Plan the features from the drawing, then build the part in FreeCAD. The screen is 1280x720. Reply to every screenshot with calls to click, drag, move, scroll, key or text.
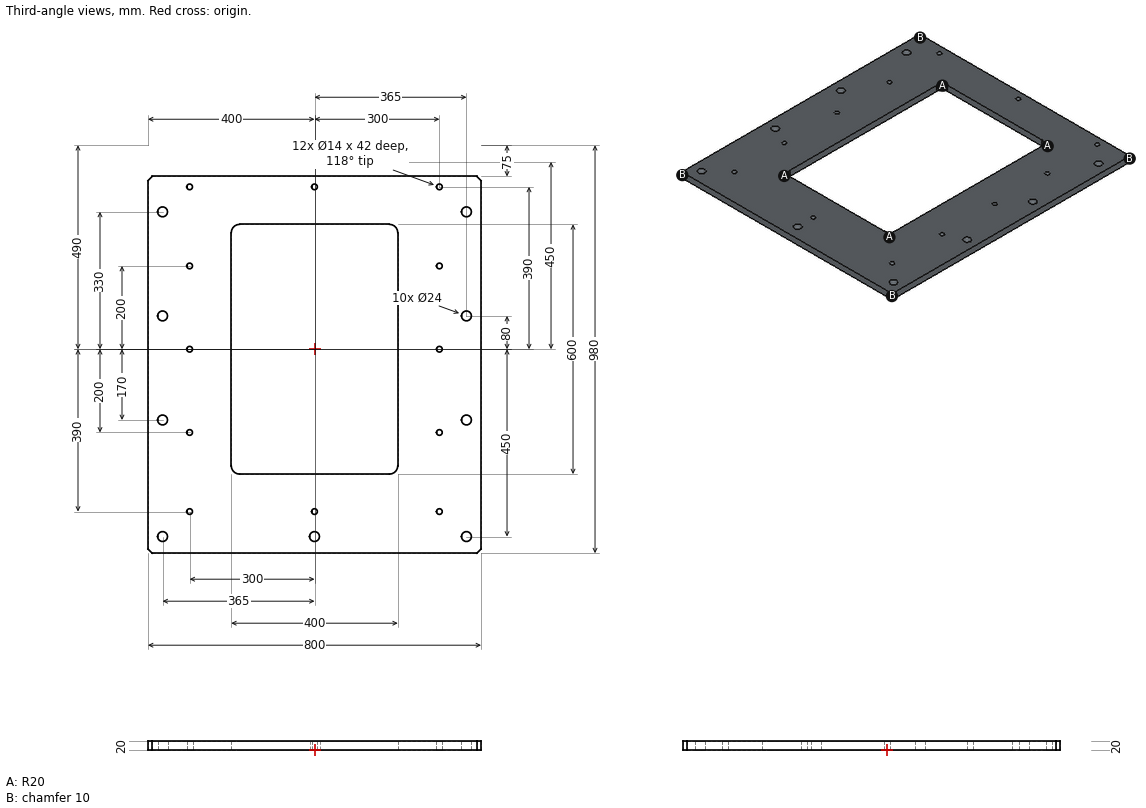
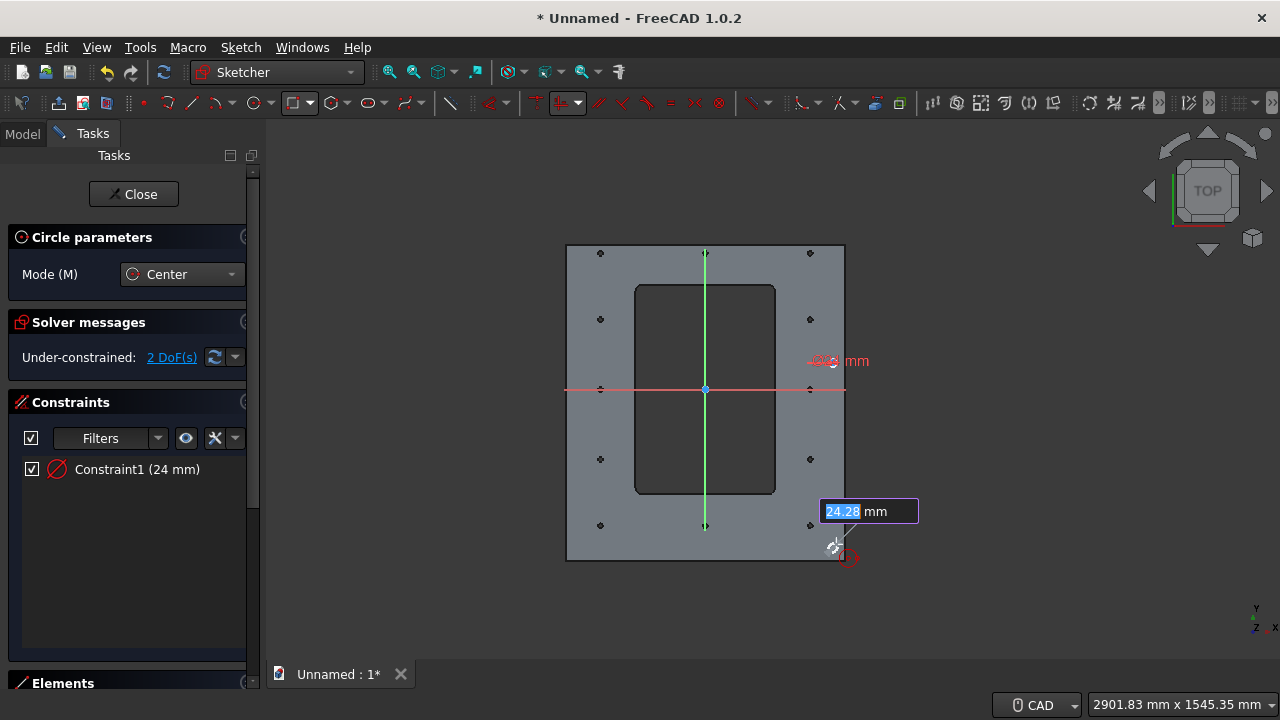
text(24)
key(Return)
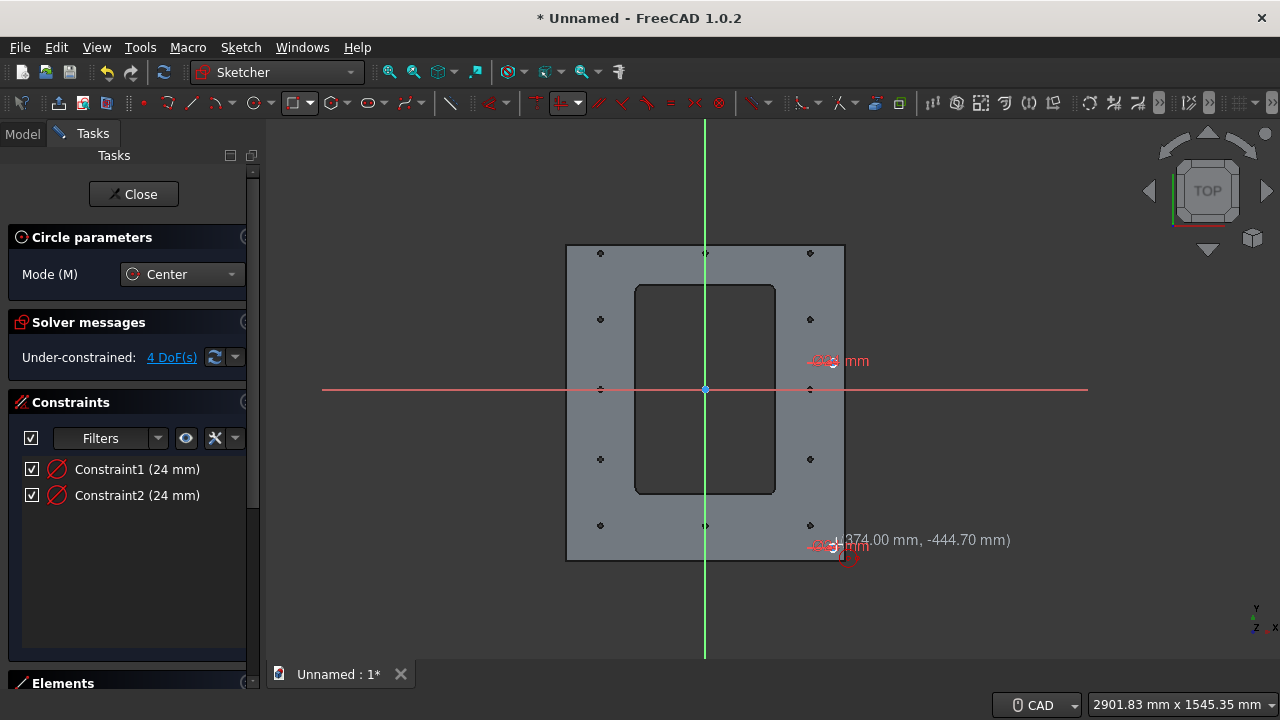
scroll(578, 547, up, 9)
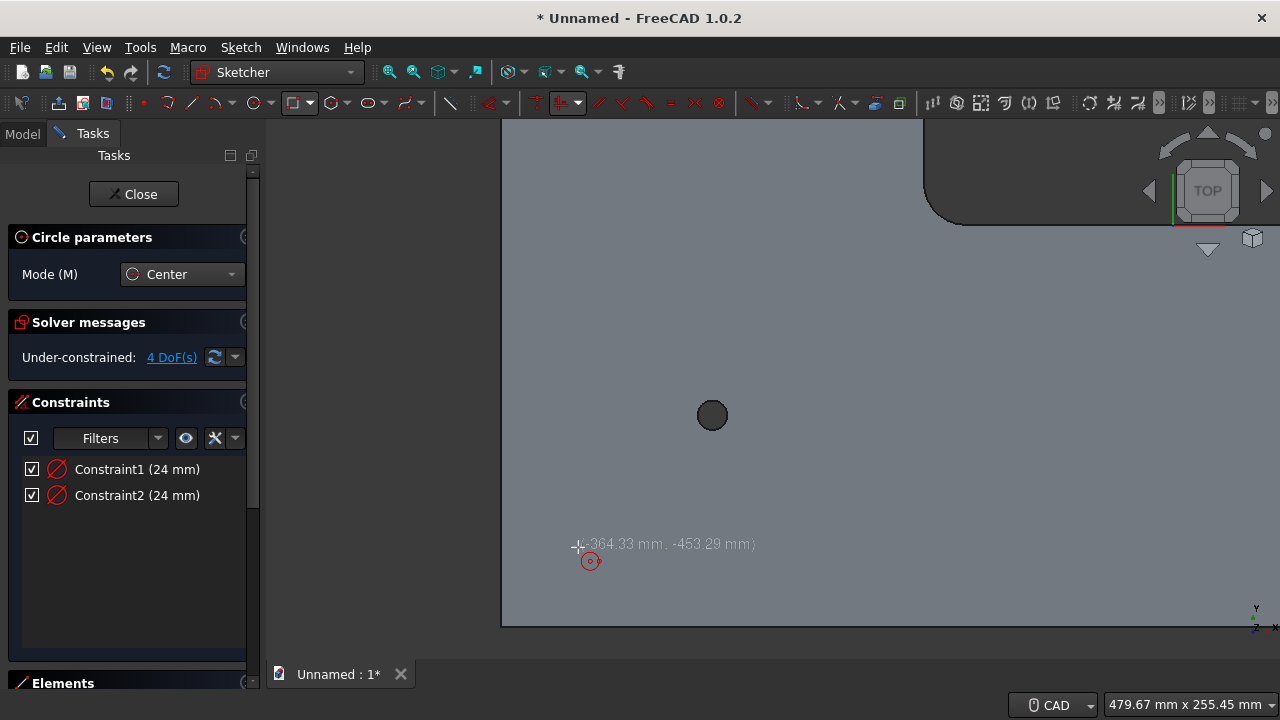
scroll(577, 547, down, 9)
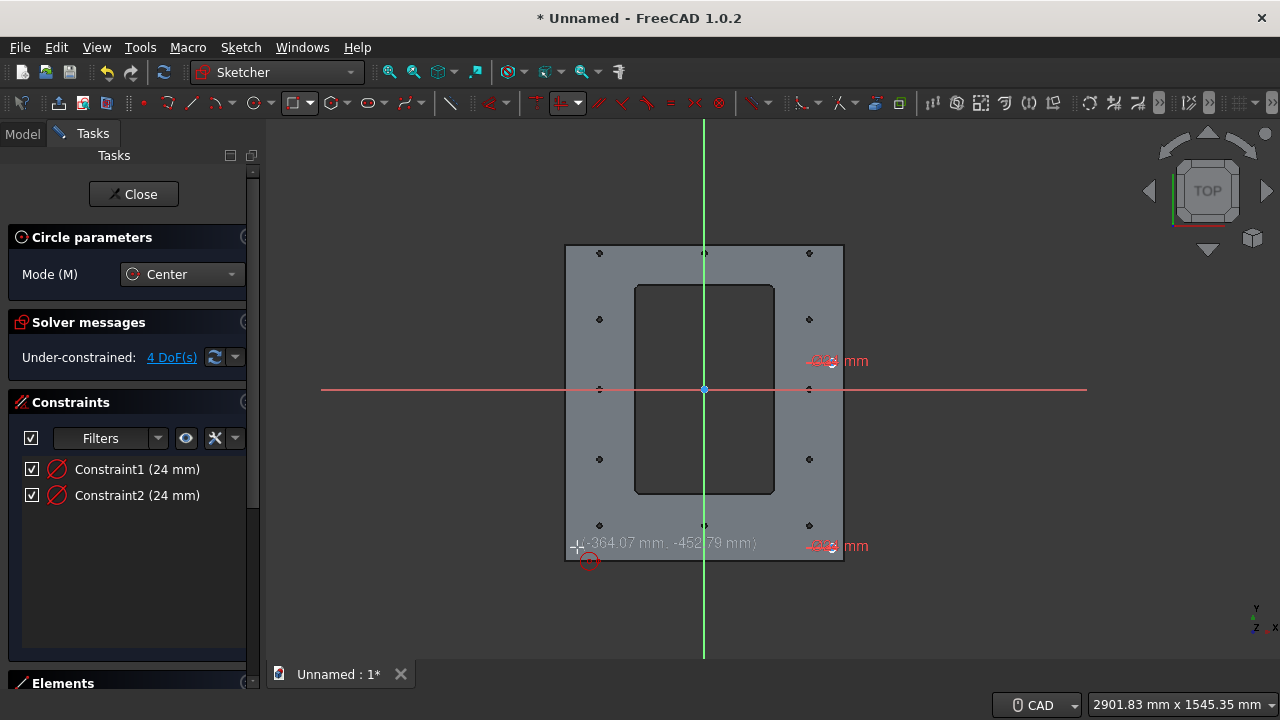
click(577, 547)
move(580, 544)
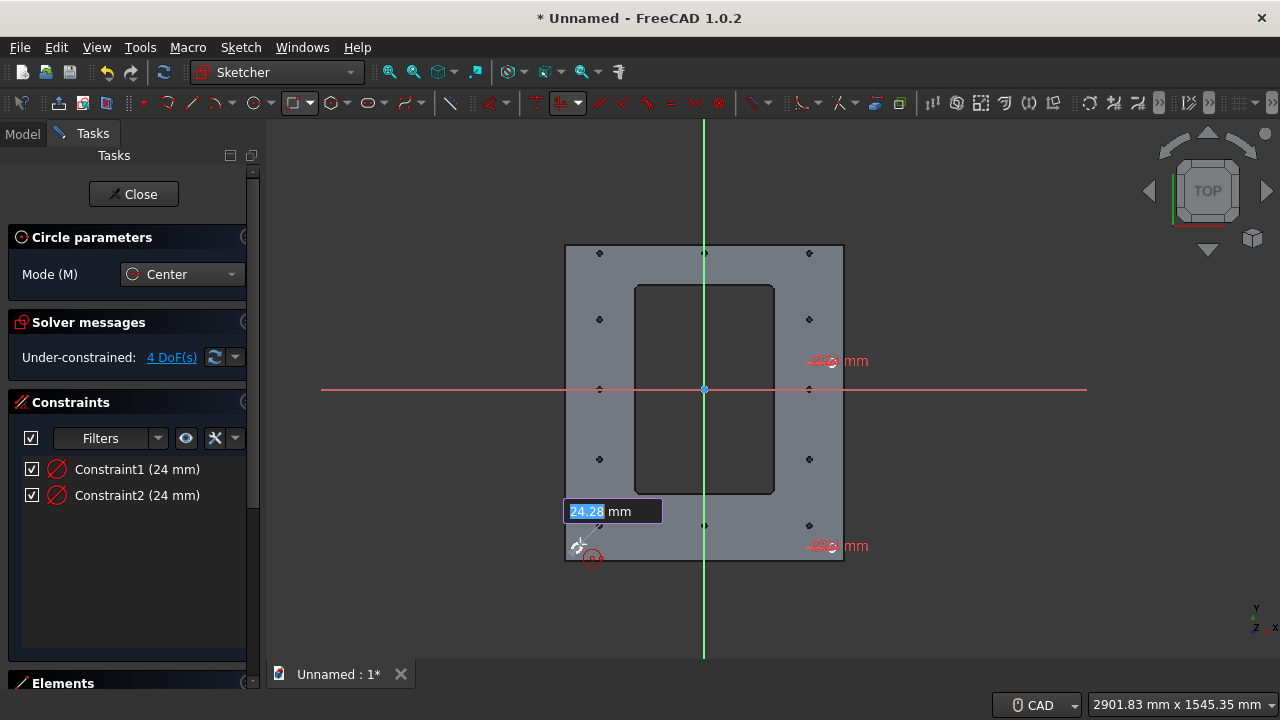
text(24)
key(Return)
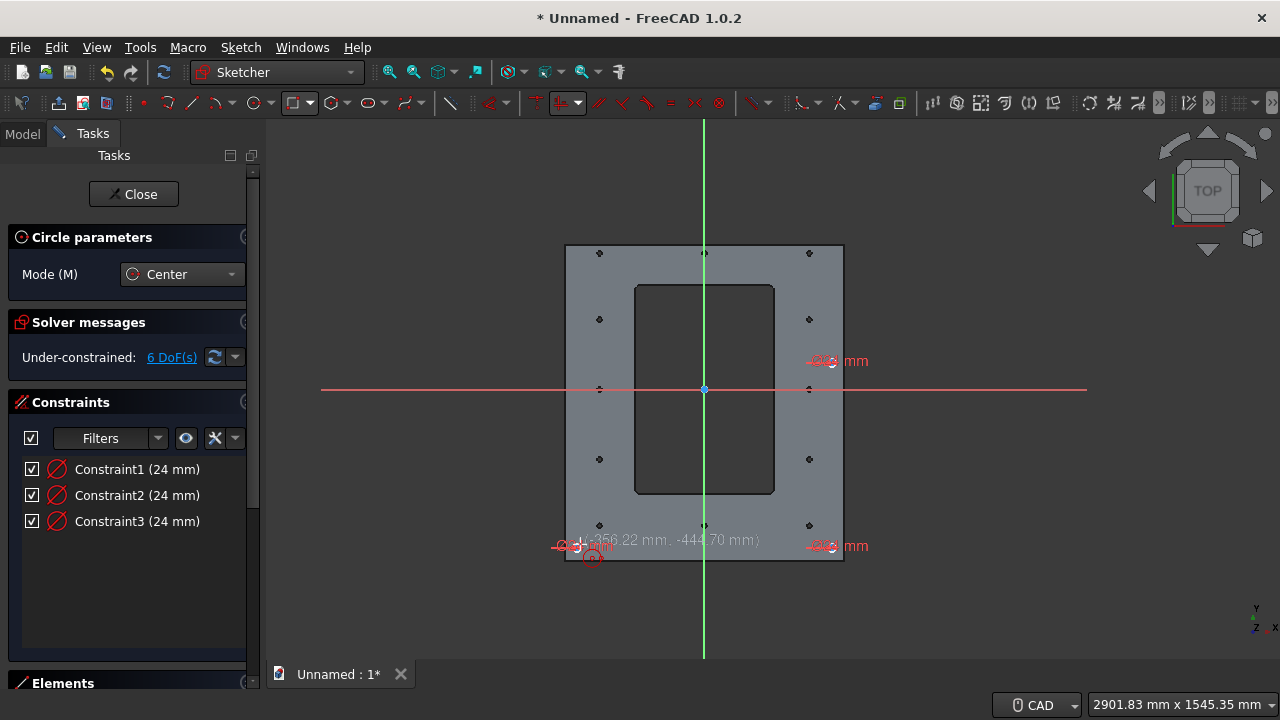
scroll(704, 547, up, 9)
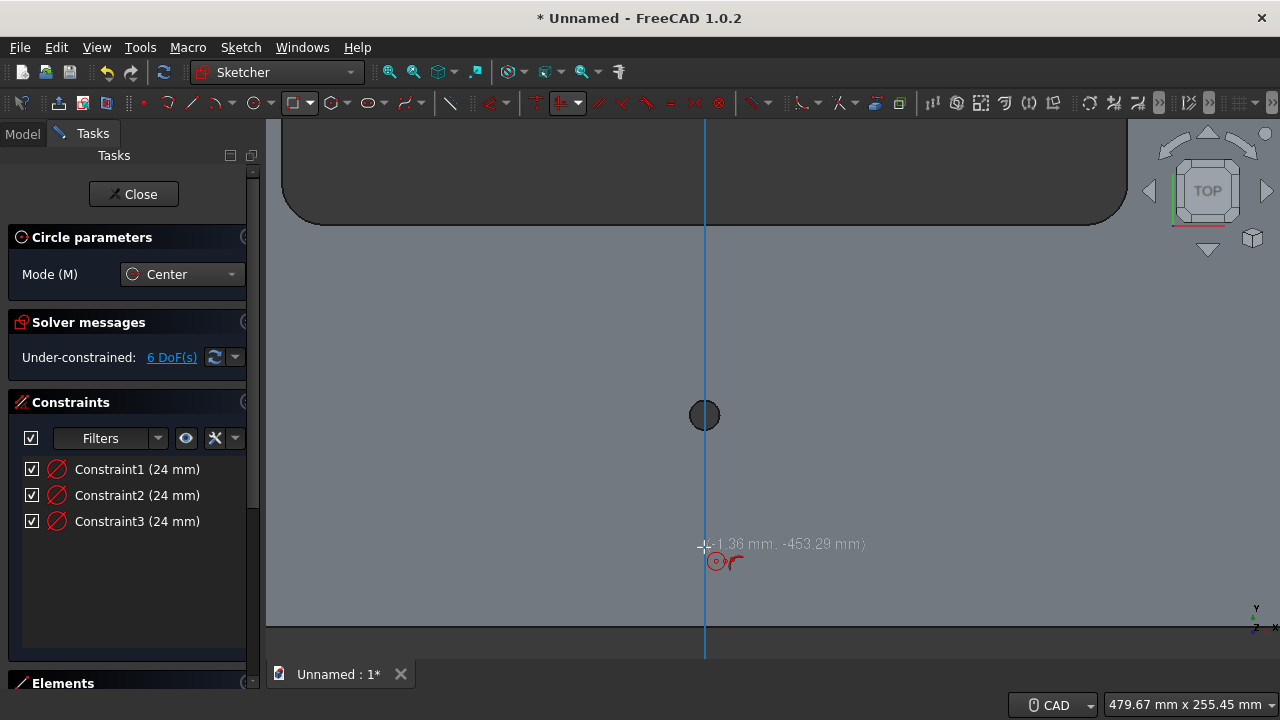
scroll(704, 547, down, 9)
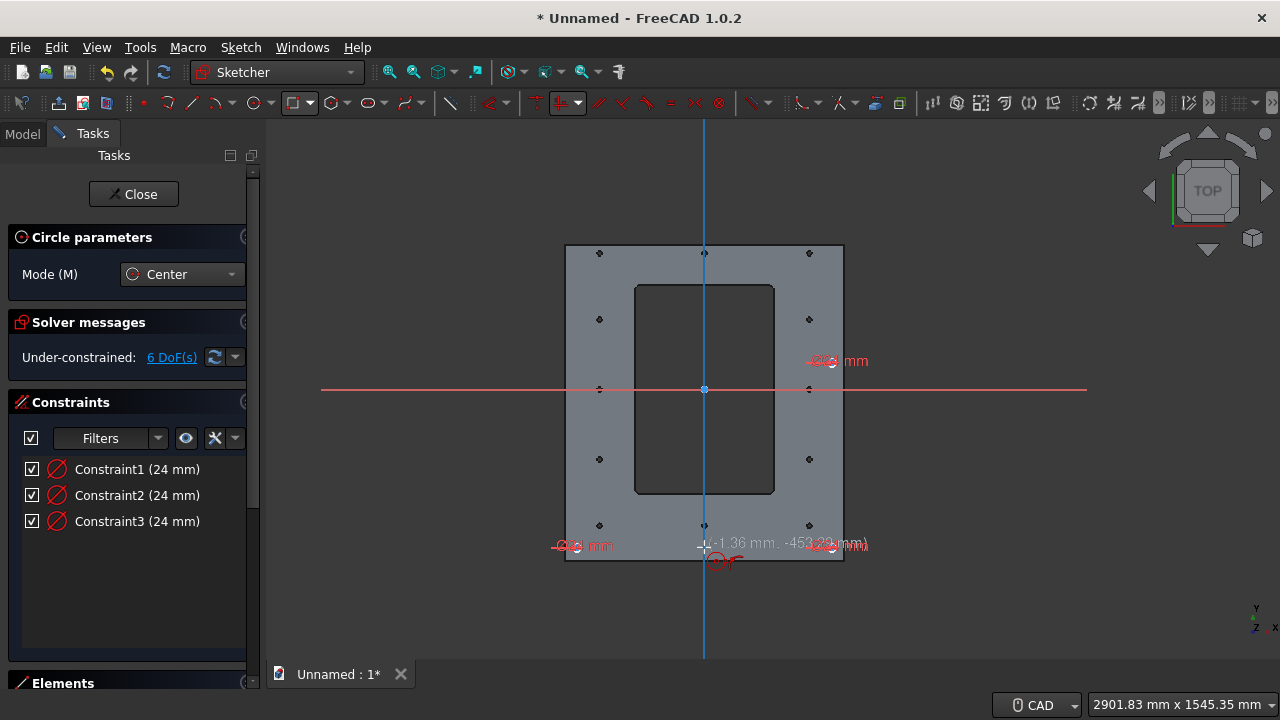
click(704, 547)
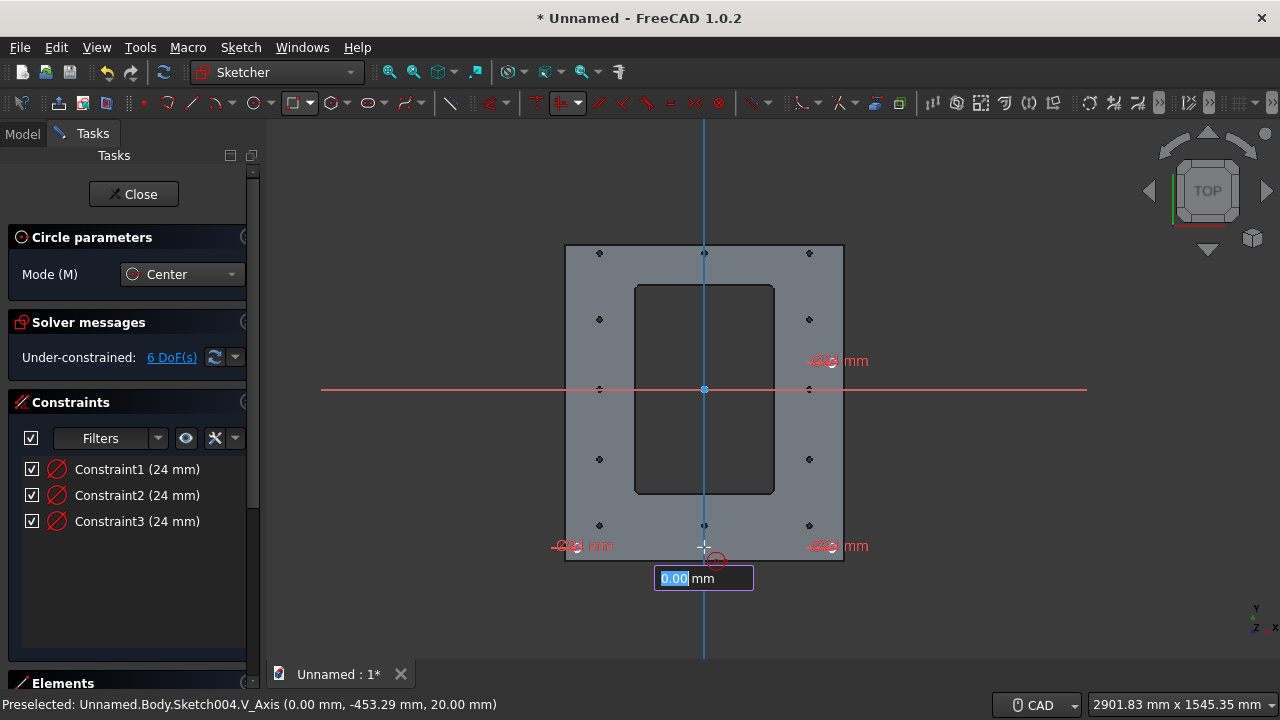
scroll(708, 545, up, 7)
move(708, 544)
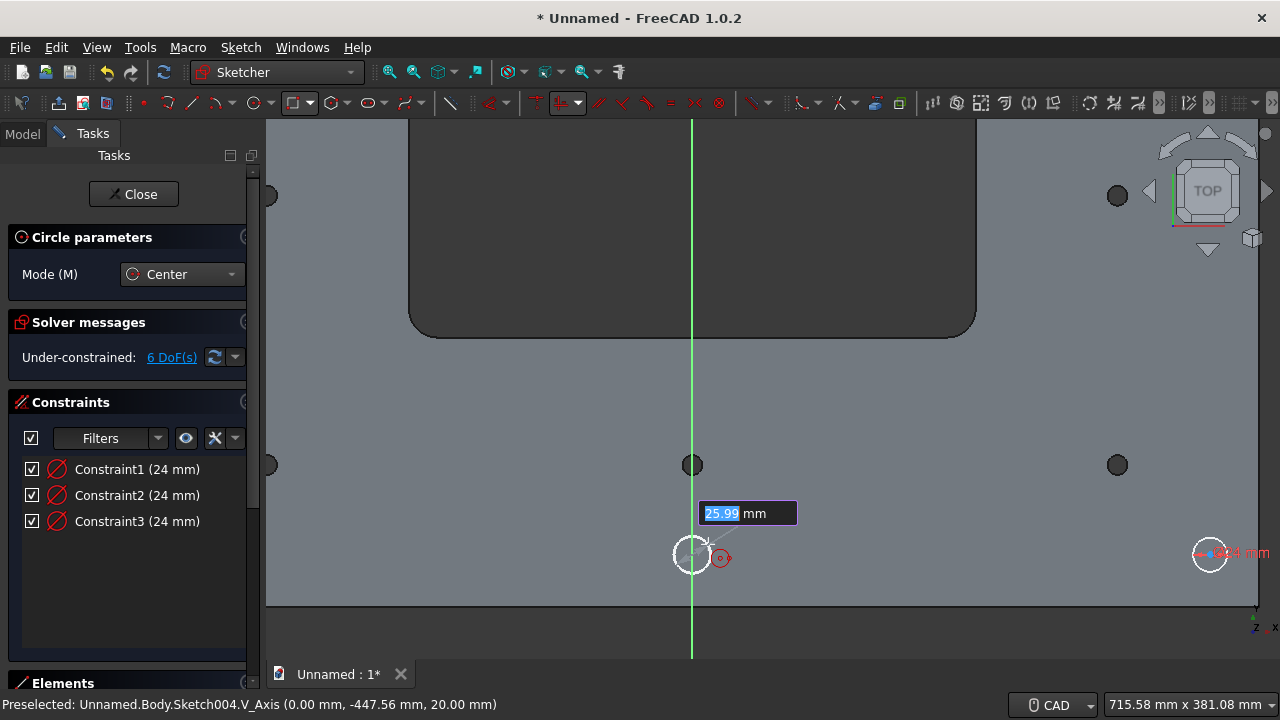
text(24)
key(Return)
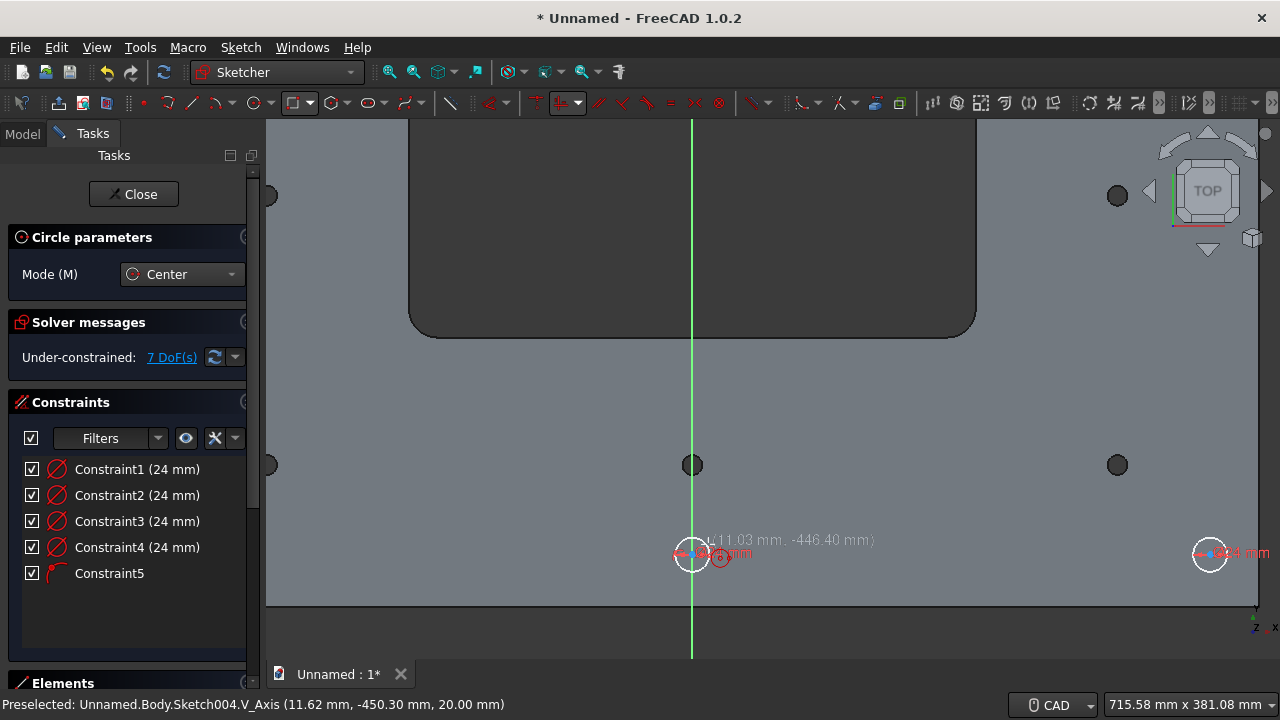
scroll(708, 545, down, 7)